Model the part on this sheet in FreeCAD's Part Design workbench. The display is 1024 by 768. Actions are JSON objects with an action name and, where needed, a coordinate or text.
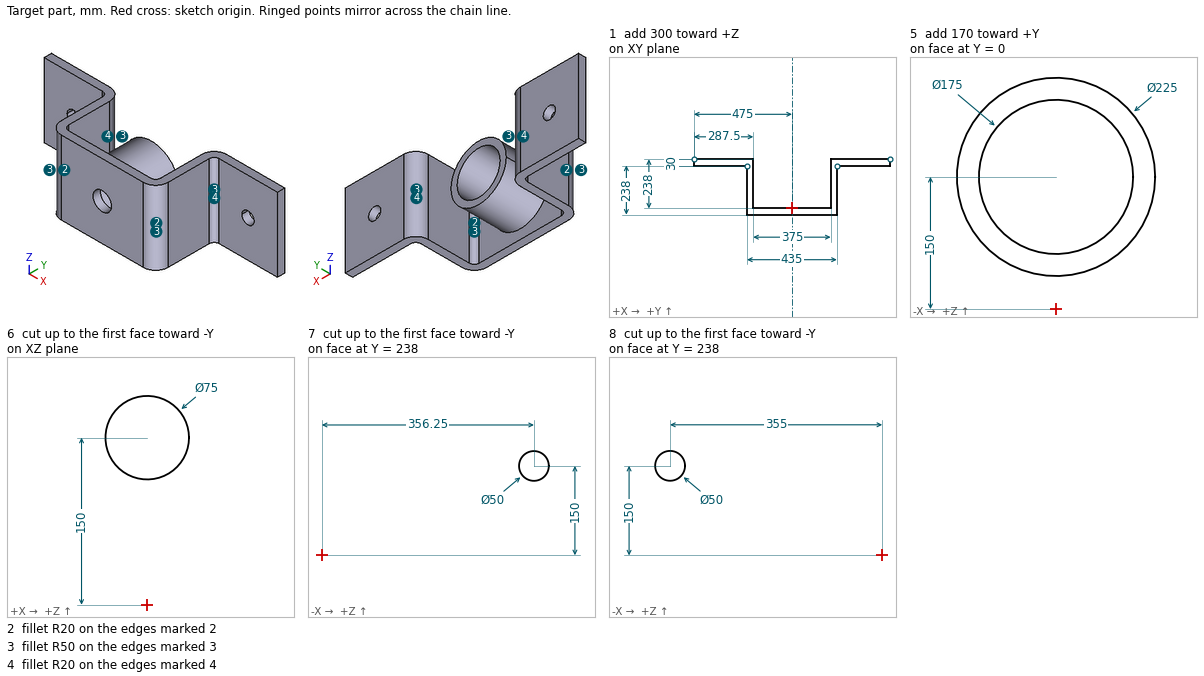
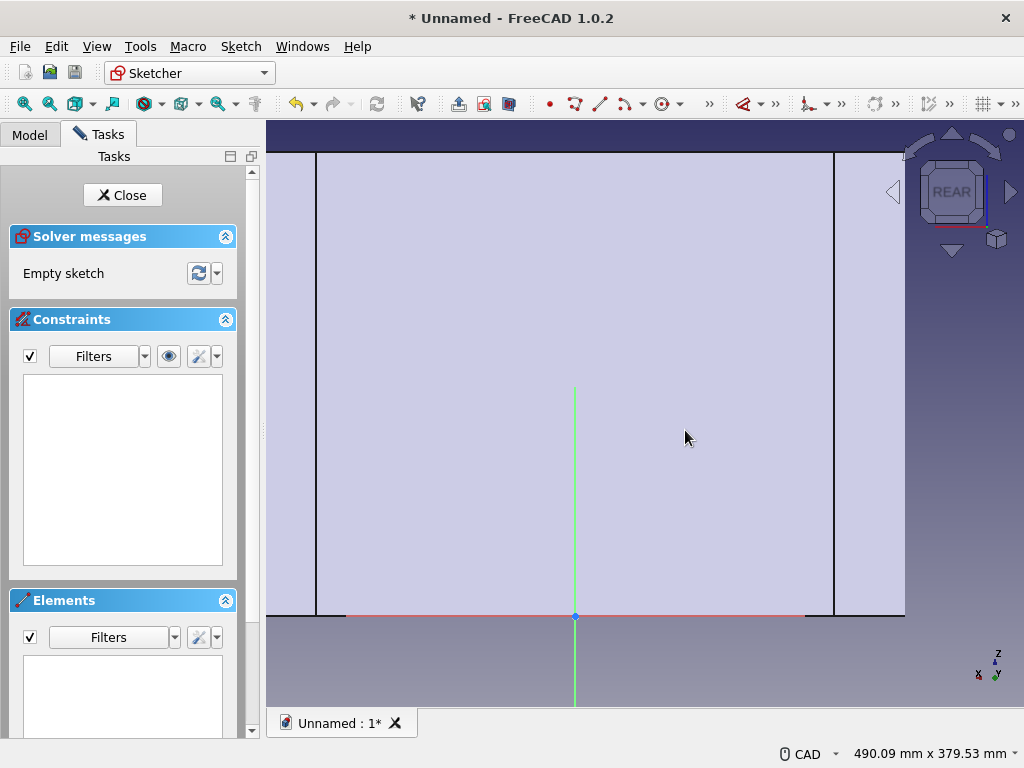
{"action": "left_click", "coordinate": [662, 104]}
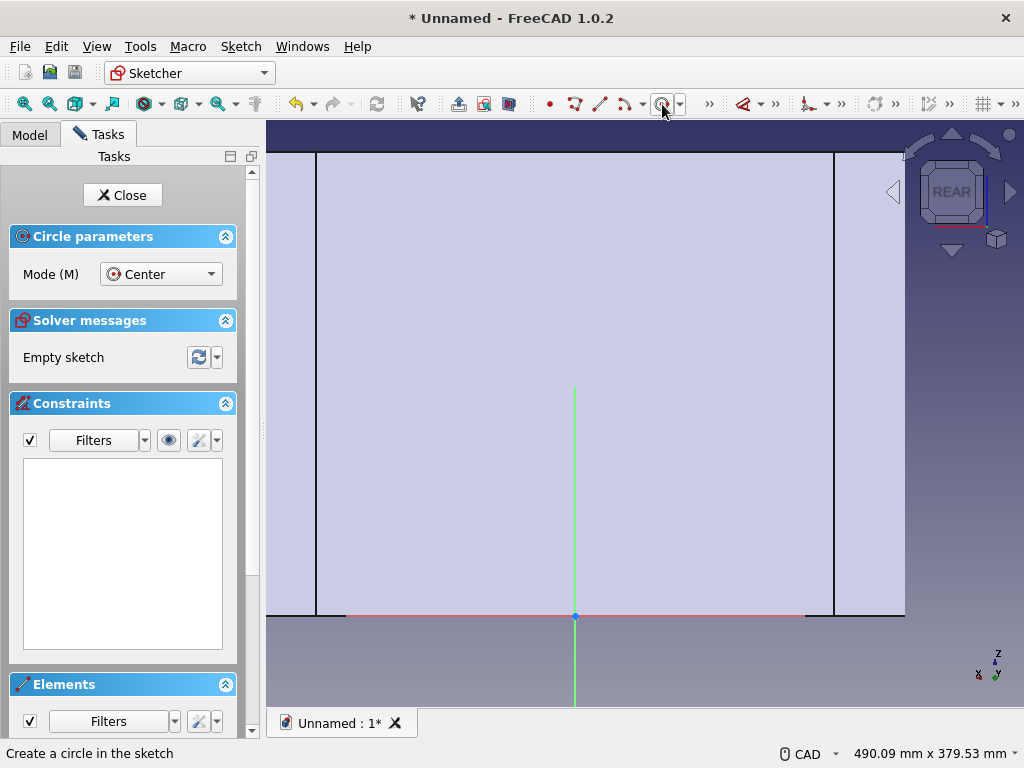
{"action": "left_click", "coordinate": [575, 384]}
{"action": "left_click", "coordinate": [698, 261]}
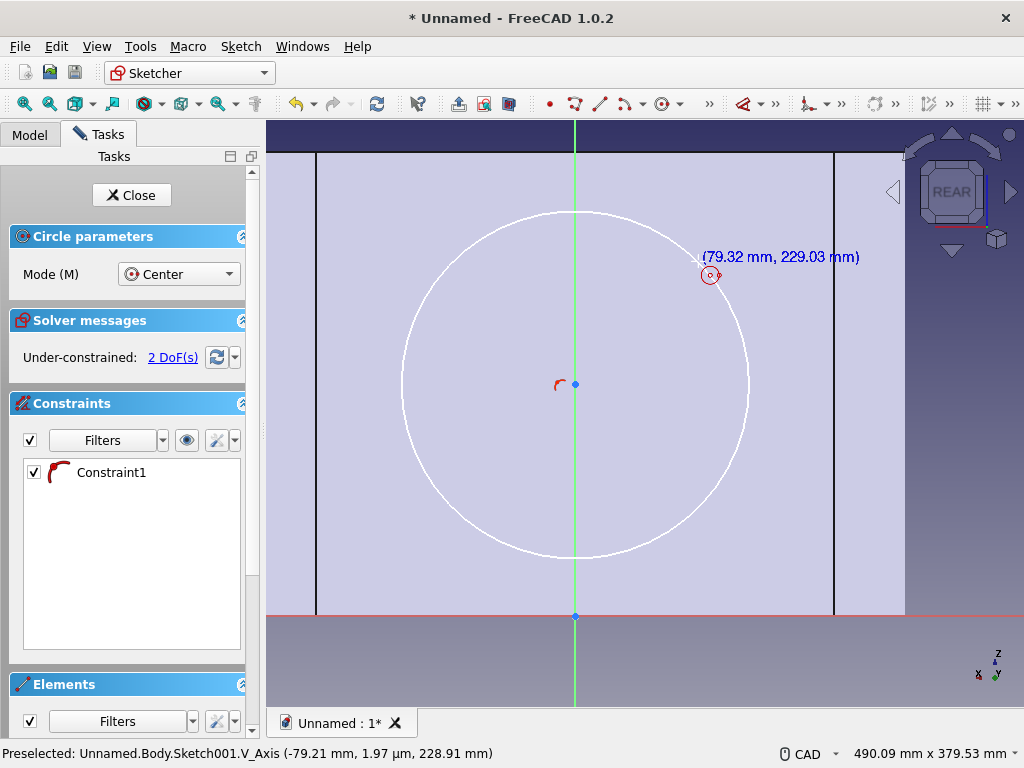
{"action": "left_click", "coordinate": [575, 385]}
{"action": "left_click", "coordinate": [671, 289]}
{"action": "key", "text": "Escape"}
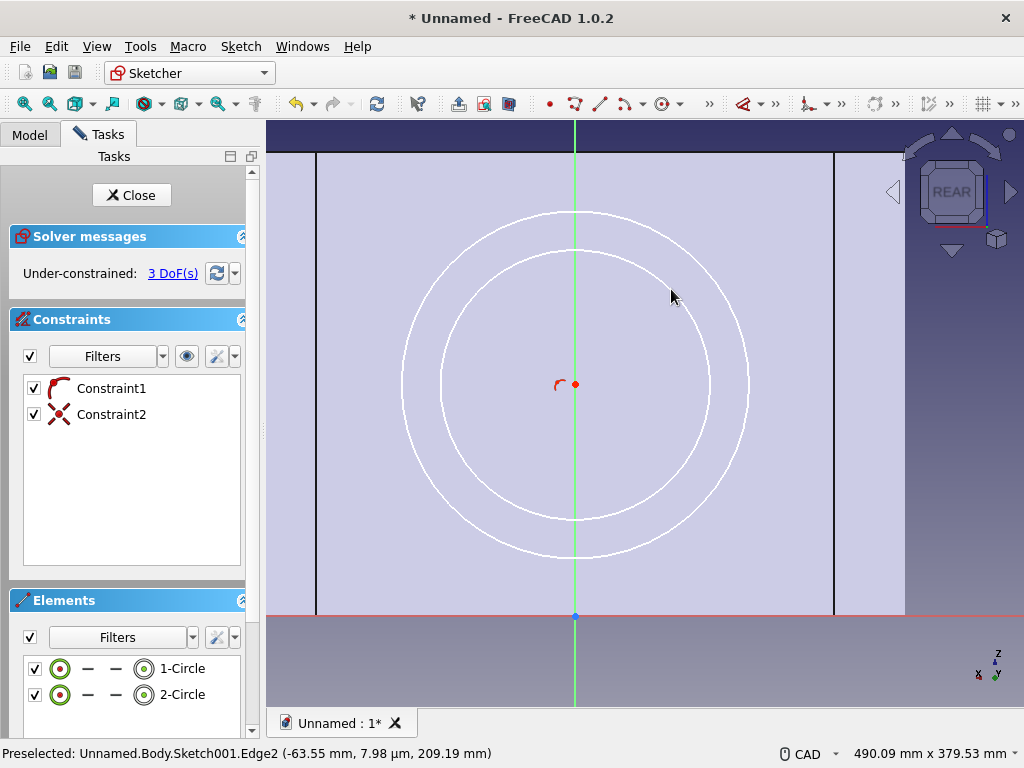
{"action": "left_click", "coordinate": [742, 104]}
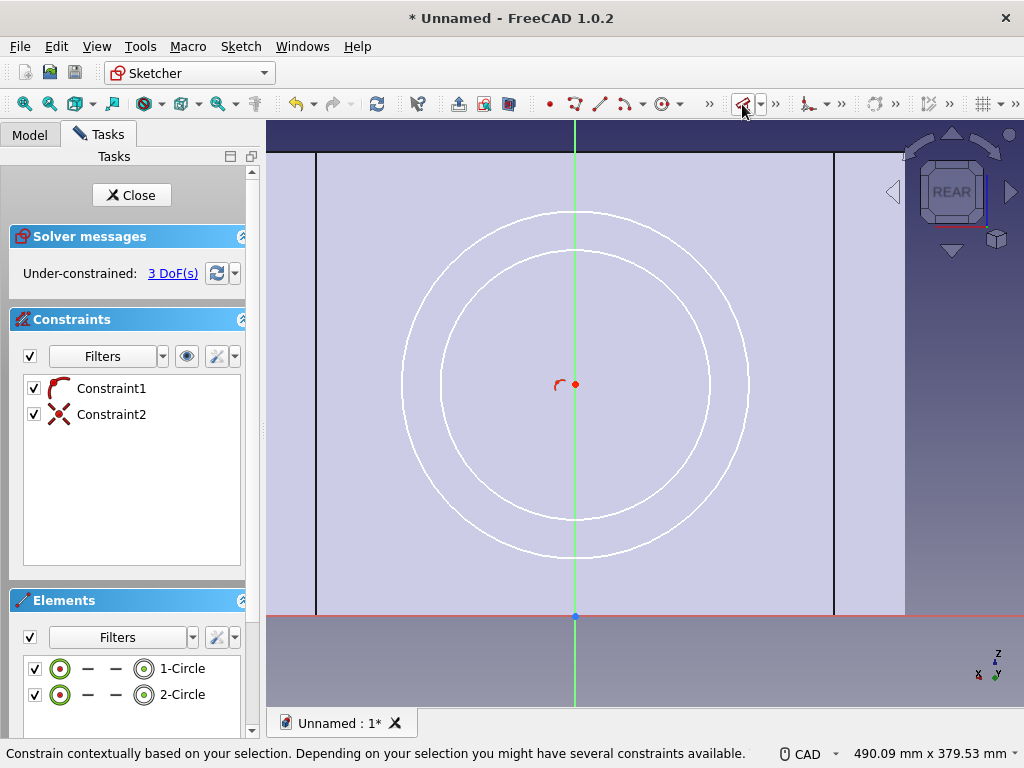
{"action": "left_click", "coordinate": [698, 262]}
{"action": "left_click", "coordinate": [721, 239]}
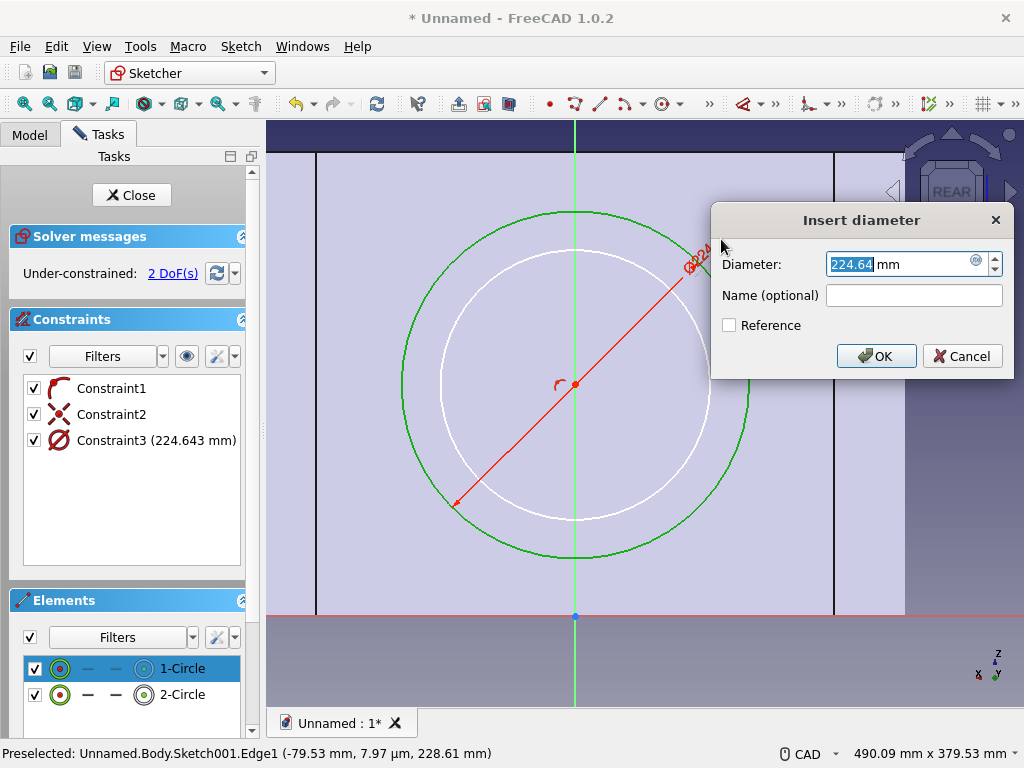
{"action": "type", "text": "225"}
{"action": "key", "text": "Return"}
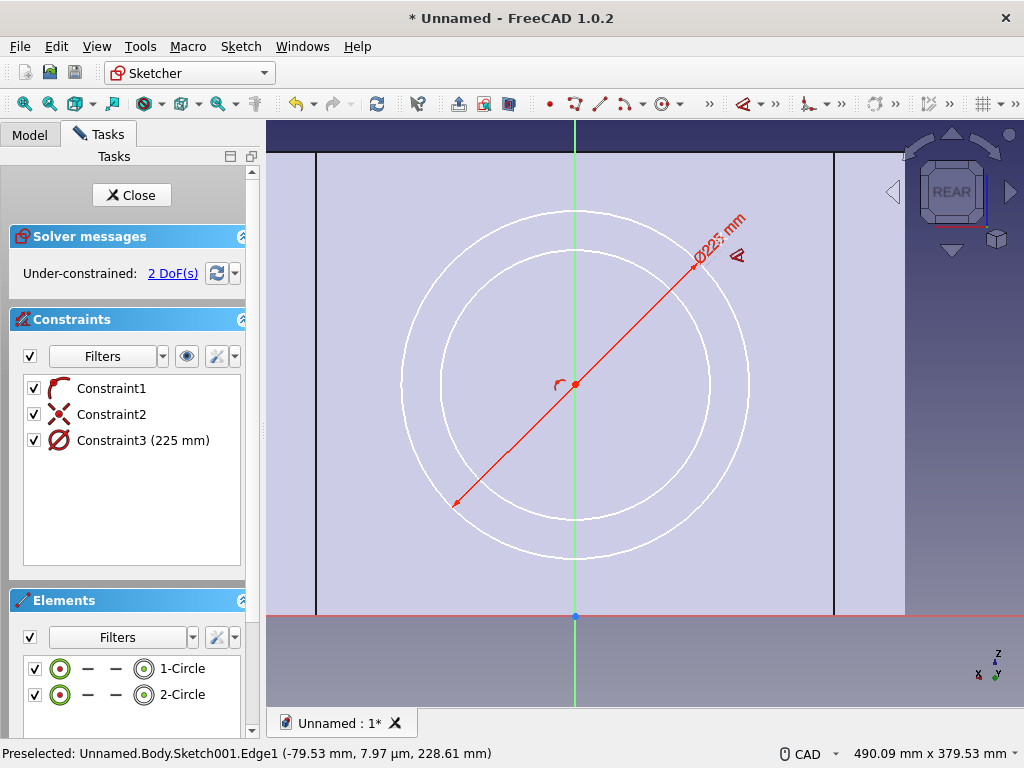
{"action": "left_click", "coordinate": [670, 289]}
{"action": "left_click", "coordinate": [757, 330]}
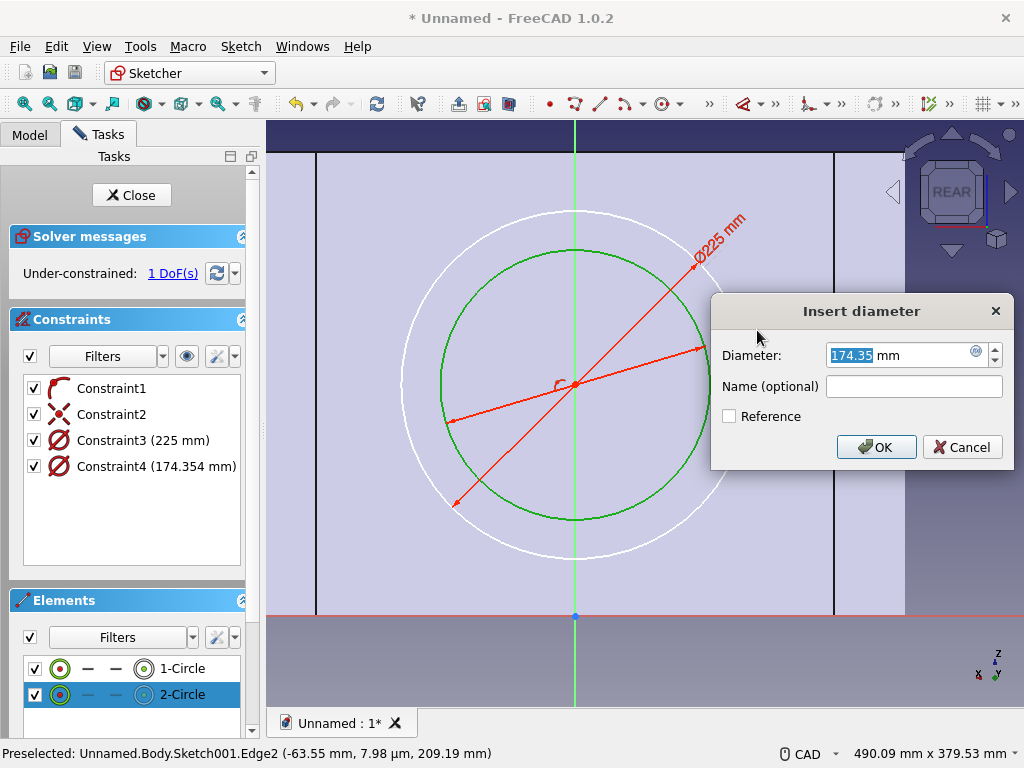
{"action": "type", "text": "175"}
{"action": "key", "text": "Return"}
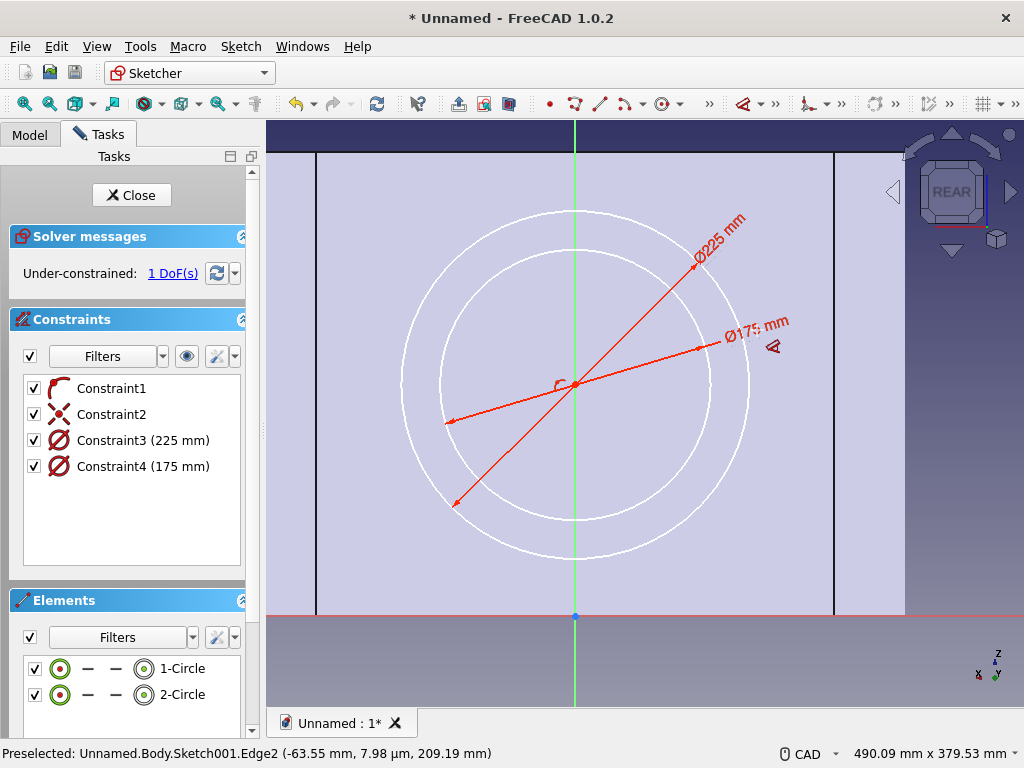
{"action": "left_click", "coordinate": [575, 385]}
{"action": "left_click", "coordinate": [609, 501]}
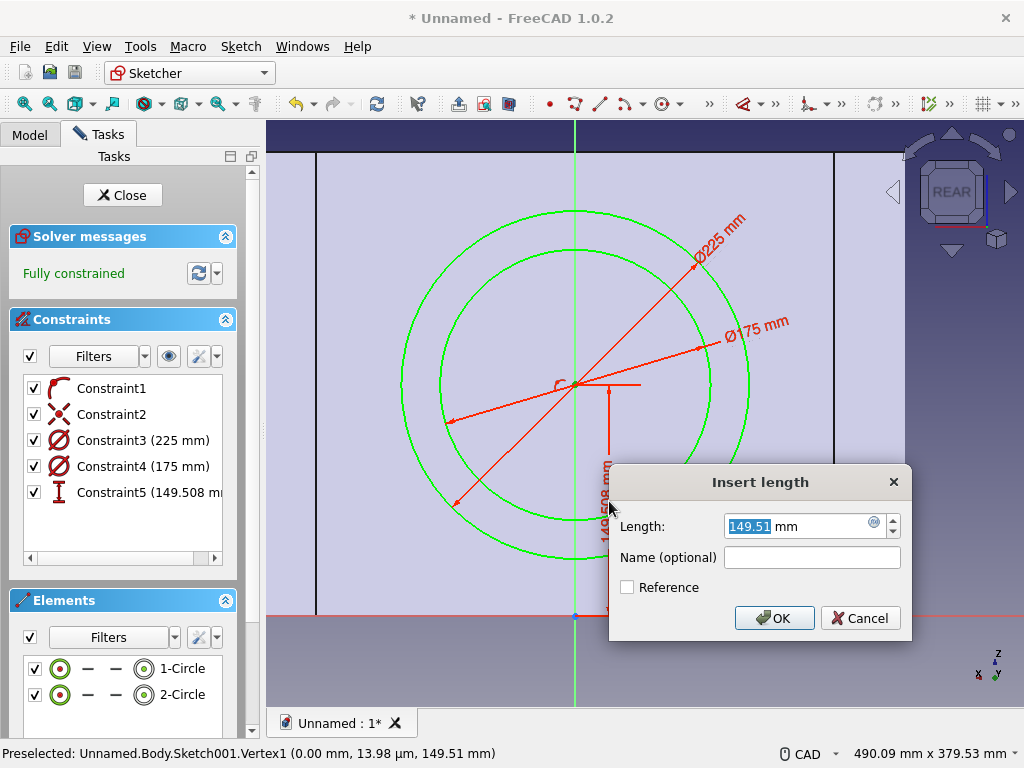
{"action": "type", "text": "150"}
{"action": "key", "text": "Return"}
{"action": "key", "text": "Escape"}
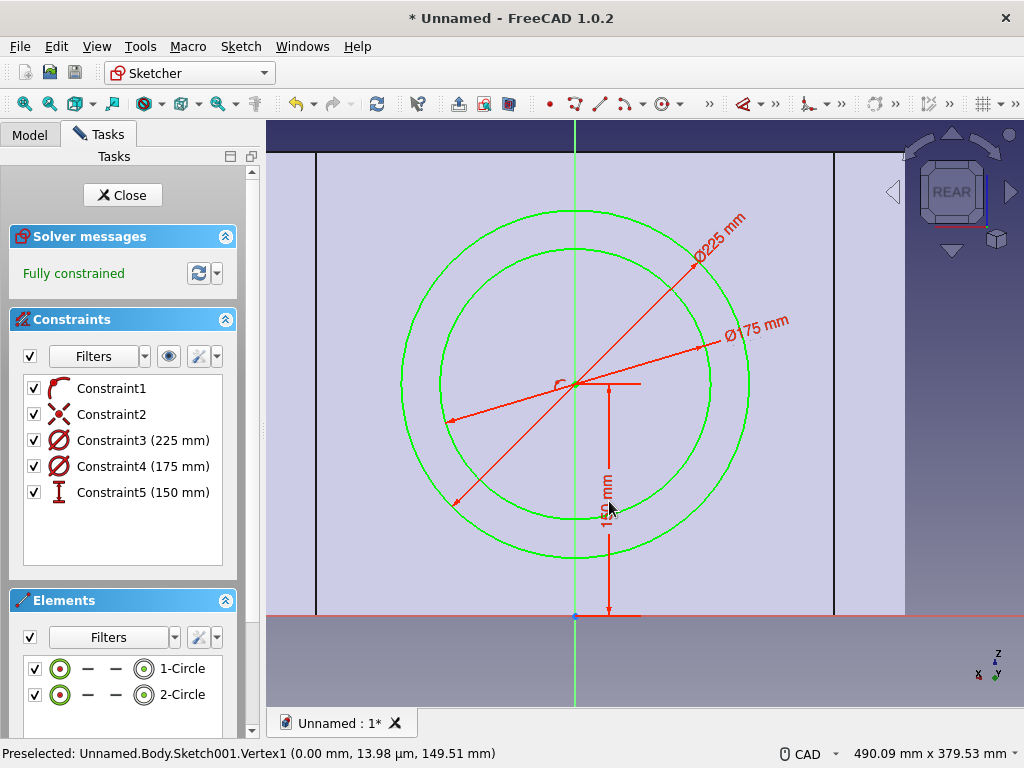
{"action": "left_click", "coordinate": [123, 195]}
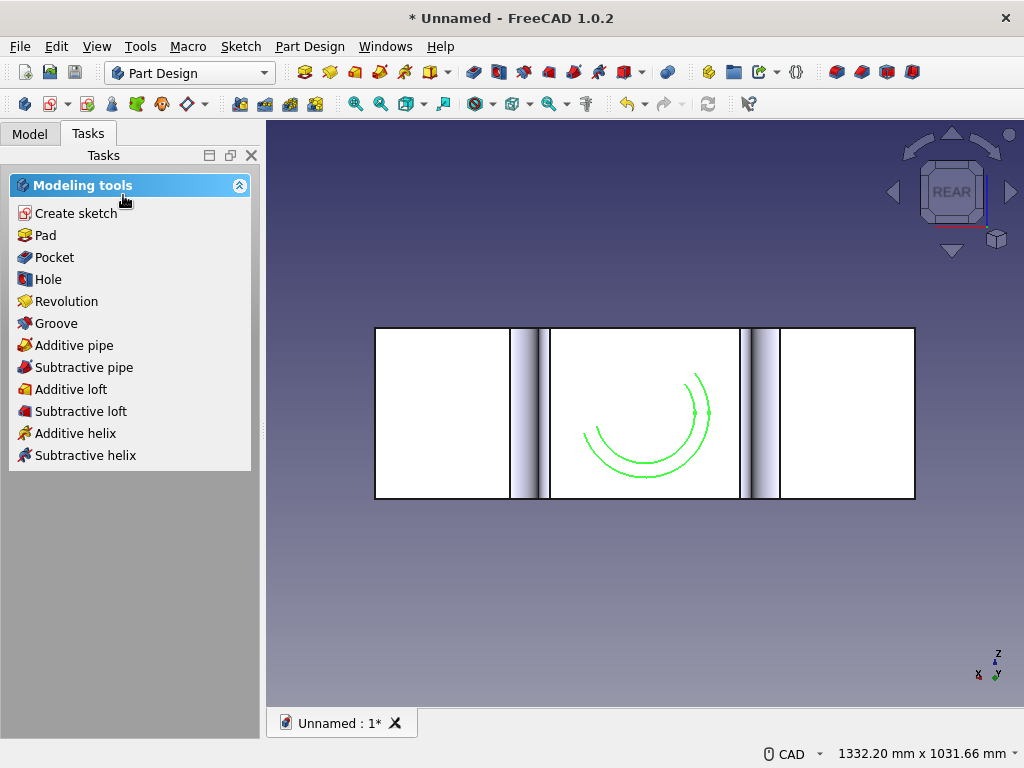
{"action": "left_click", "coordinate": [305, 72]}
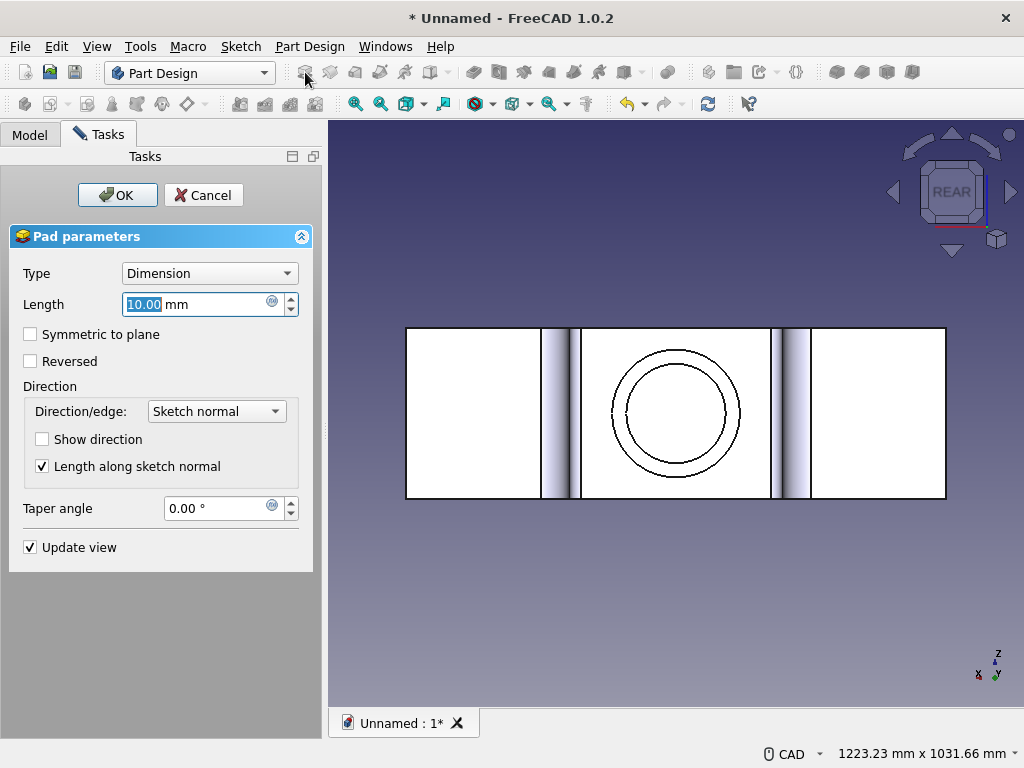
{"action": "type", "text": "170"}
{"action": "key", "text": "Tab"}